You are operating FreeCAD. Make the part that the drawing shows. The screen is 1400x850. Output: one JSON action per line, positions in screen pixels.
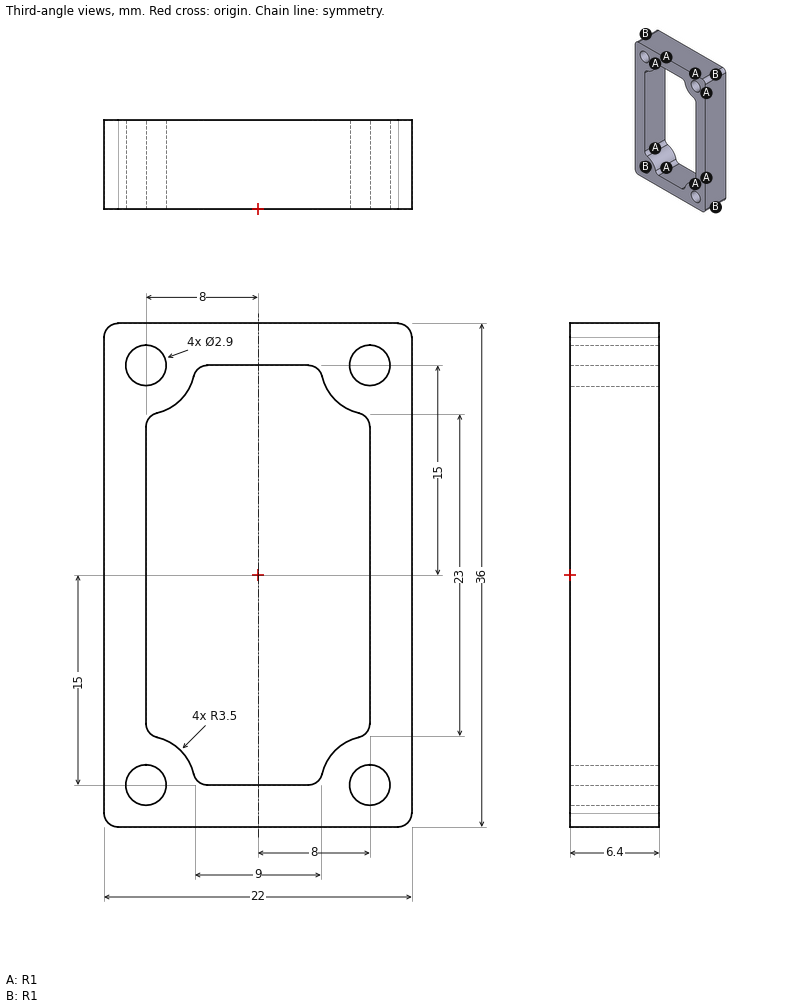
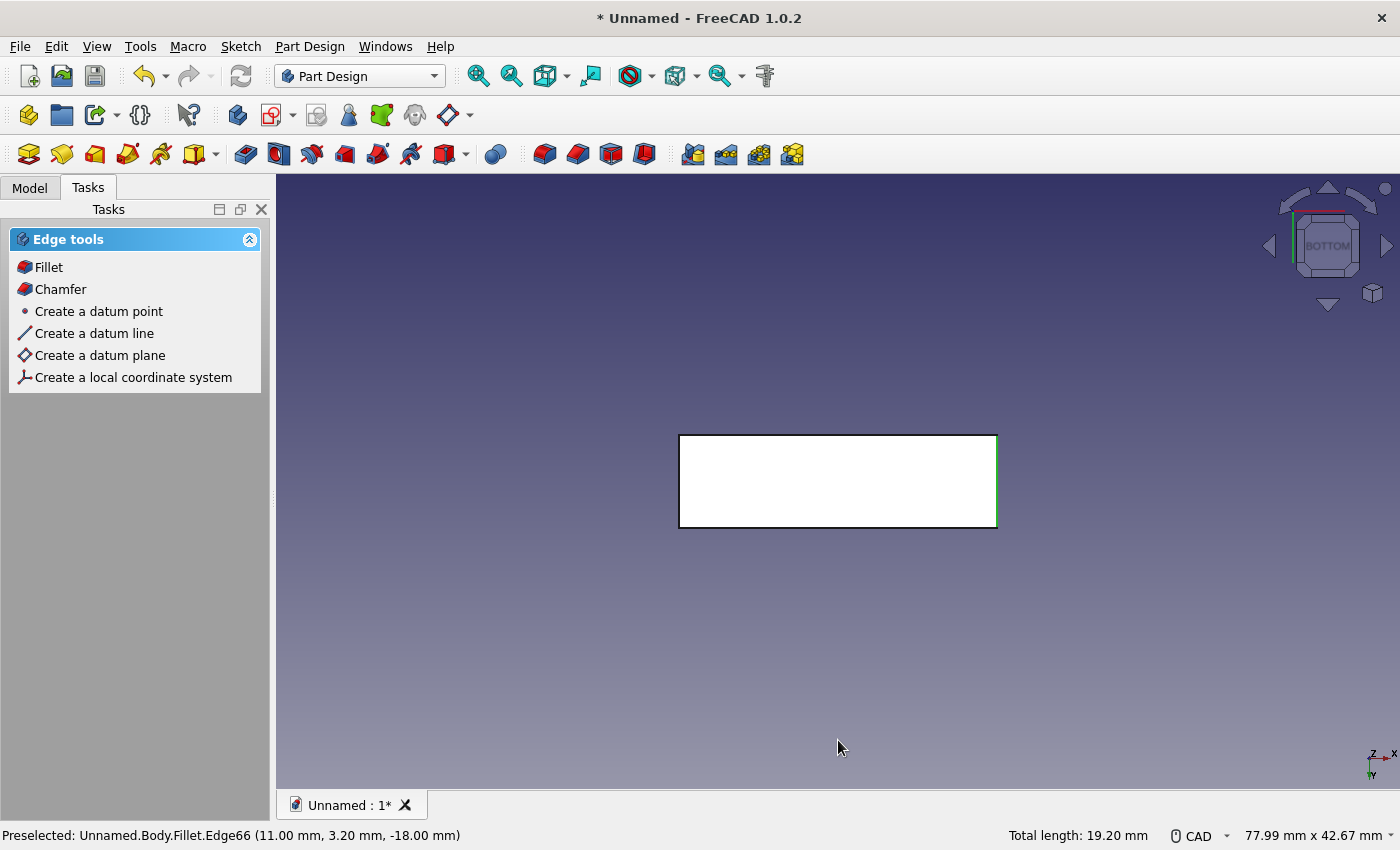
{"action": "left_click", "coordinate": [479, 76]}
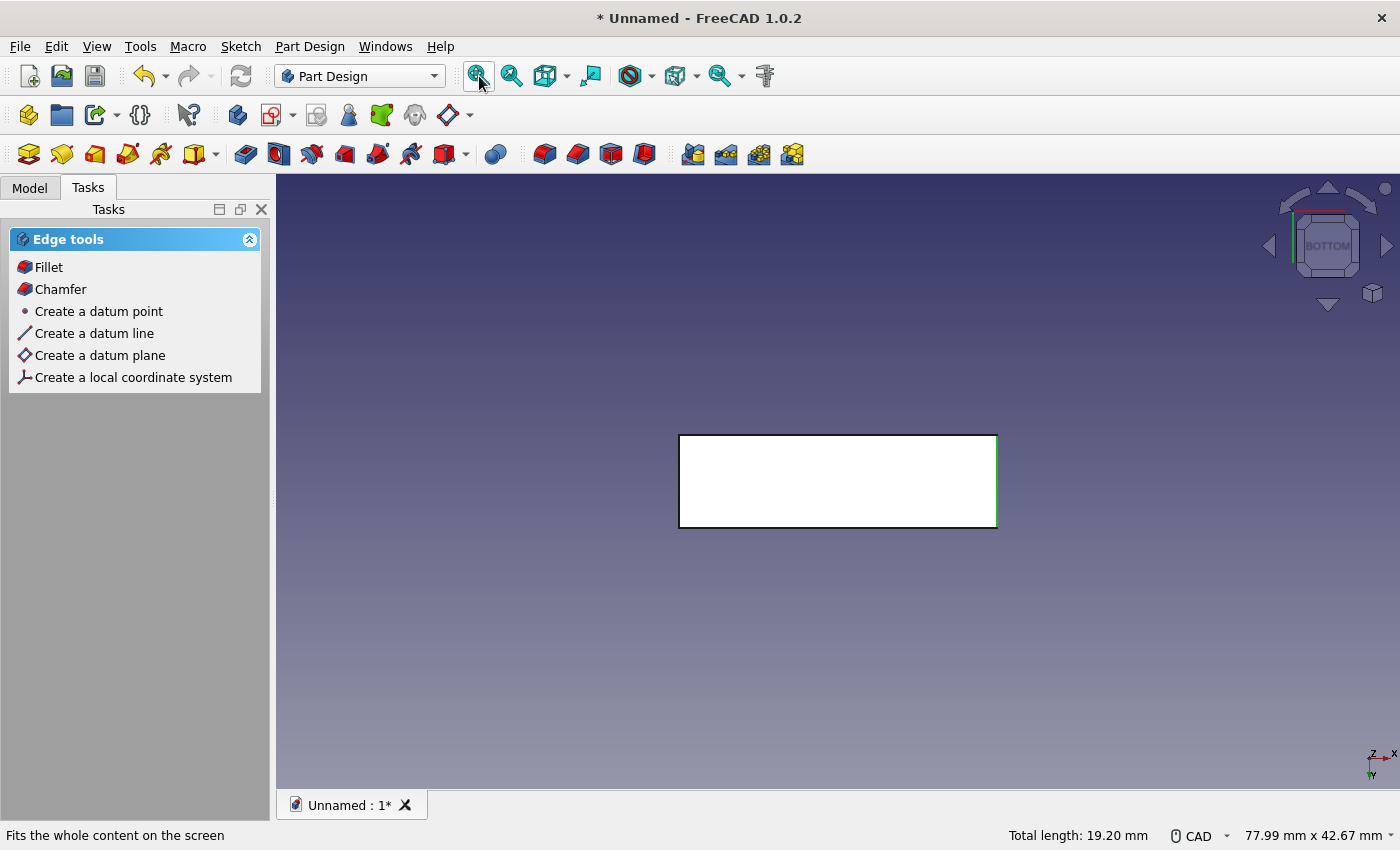
{"action": "left_click", "coordinate": [679, 480], "text": "ctrl"}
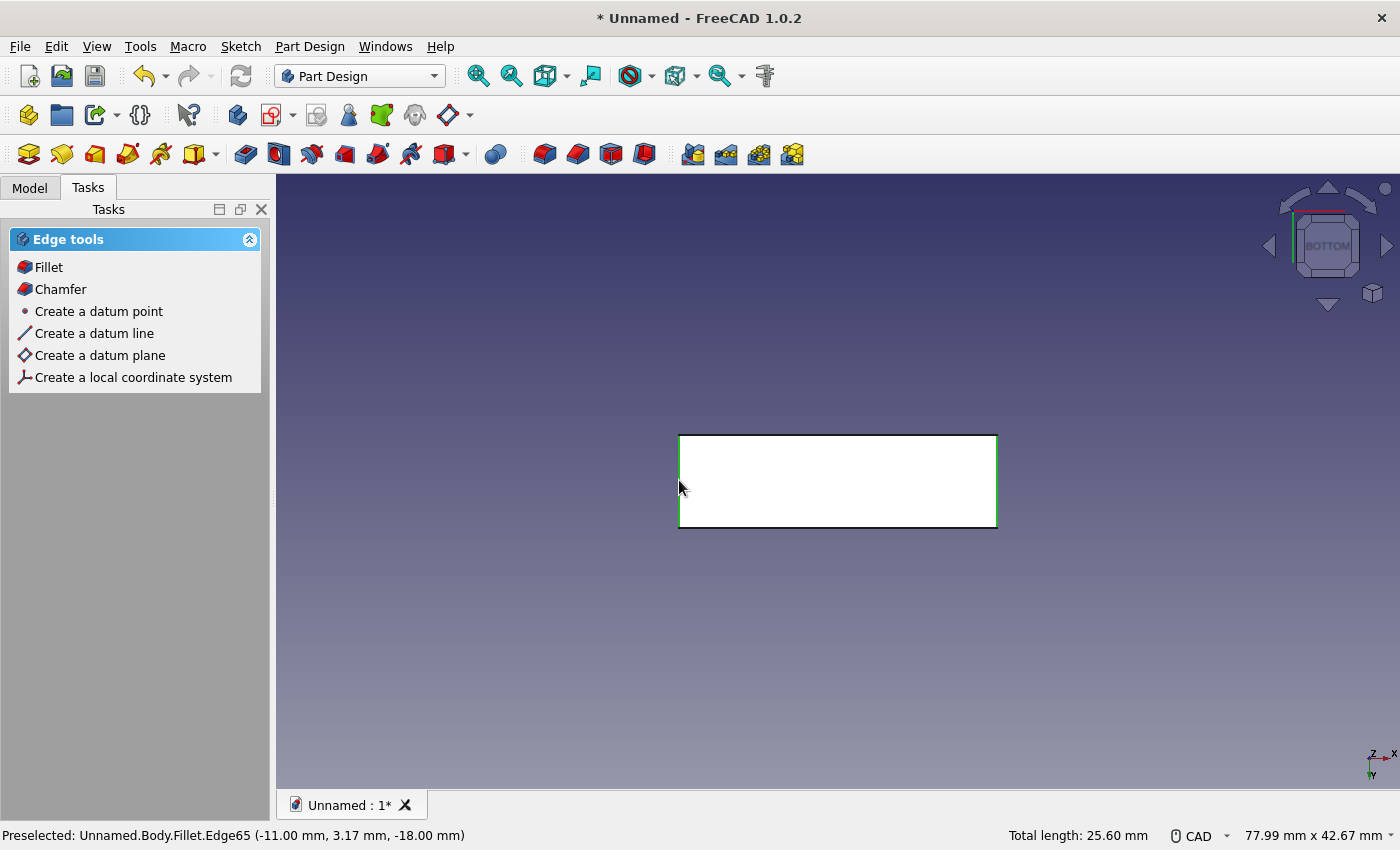
{"action": "left_click", "coordinate": [545, 154]}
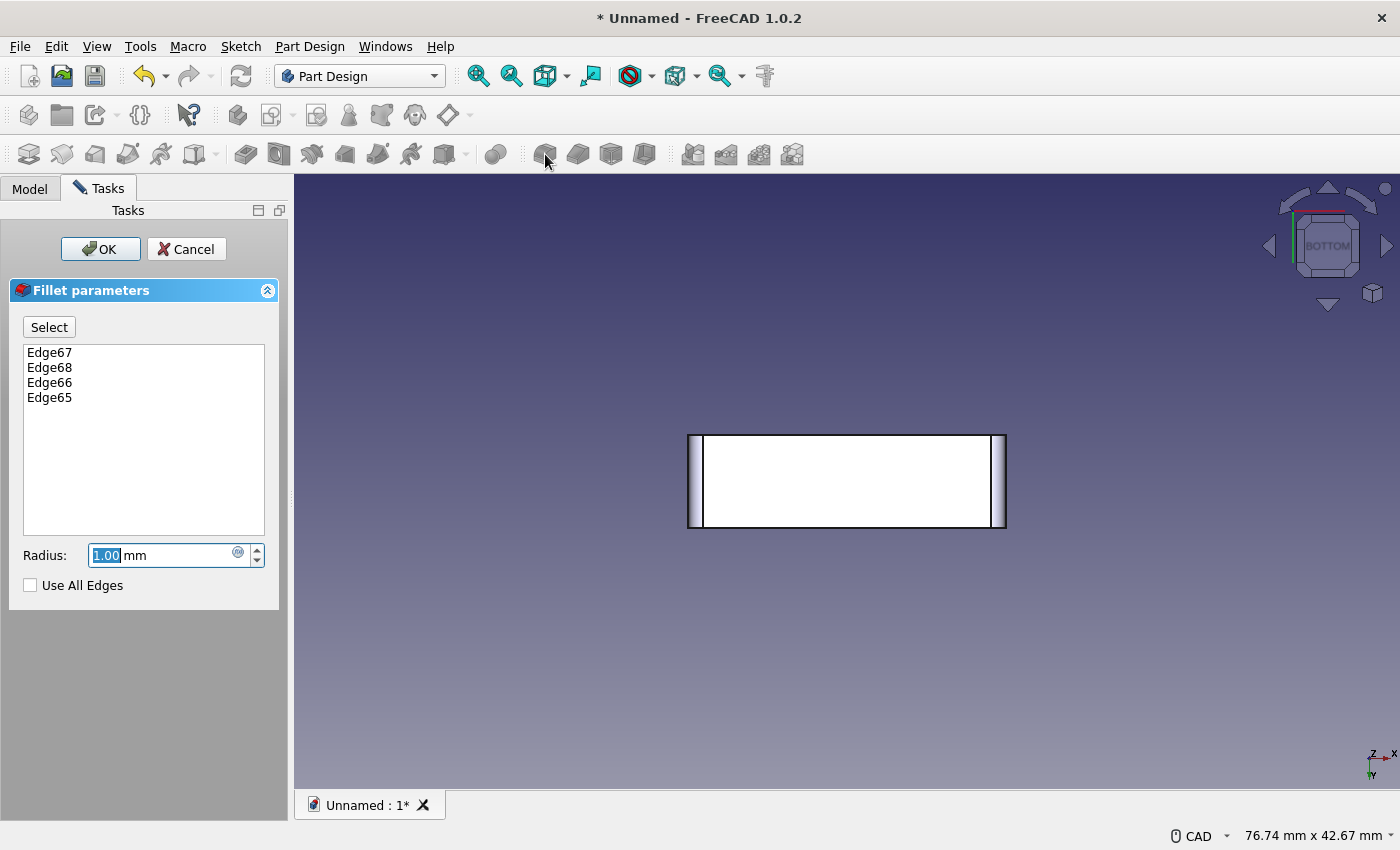
{"action": "type", "text": "1"}
{"action": "key", "text": "Tab"}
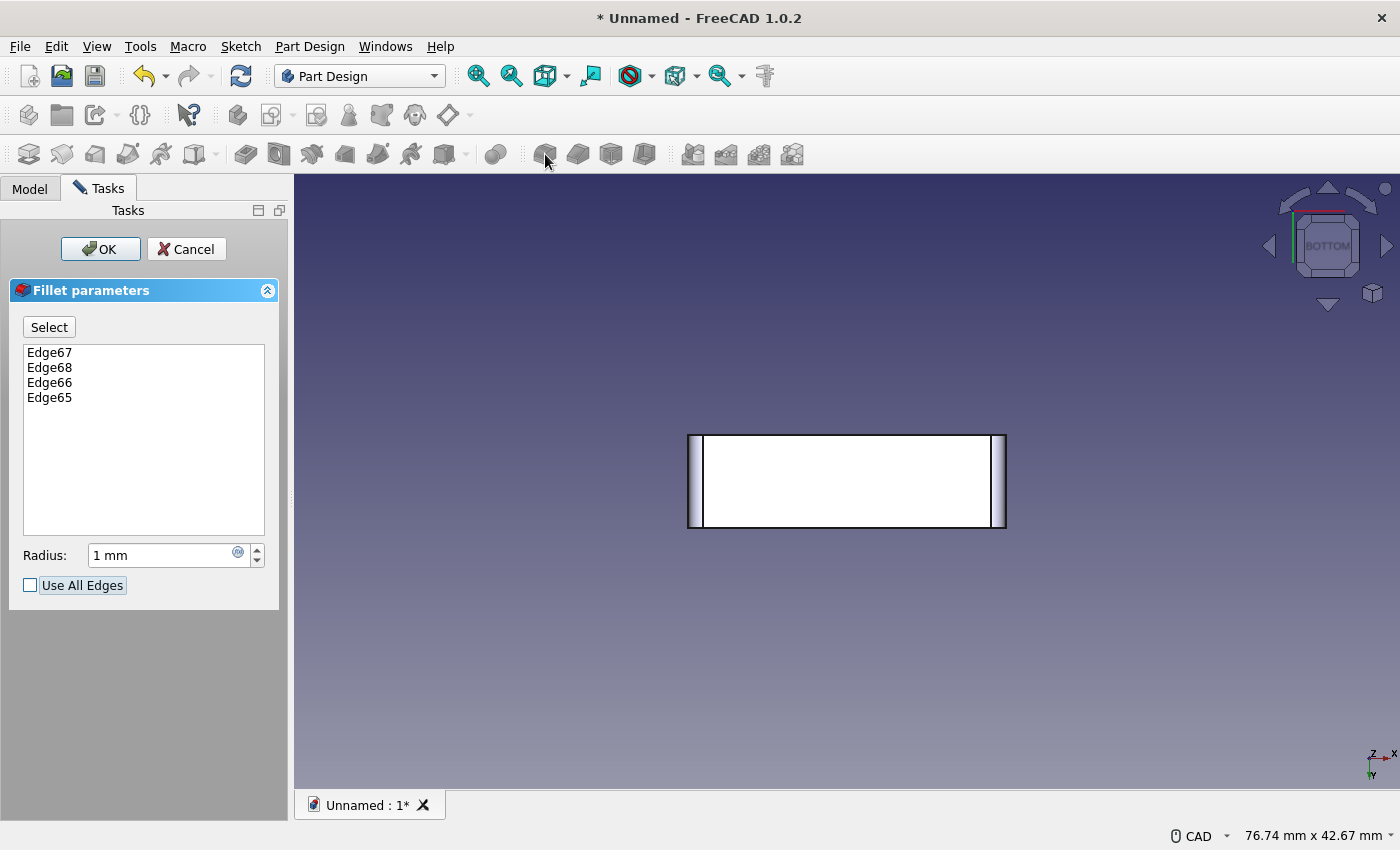
{"action": "left_click", "coordinate": [101, 249]}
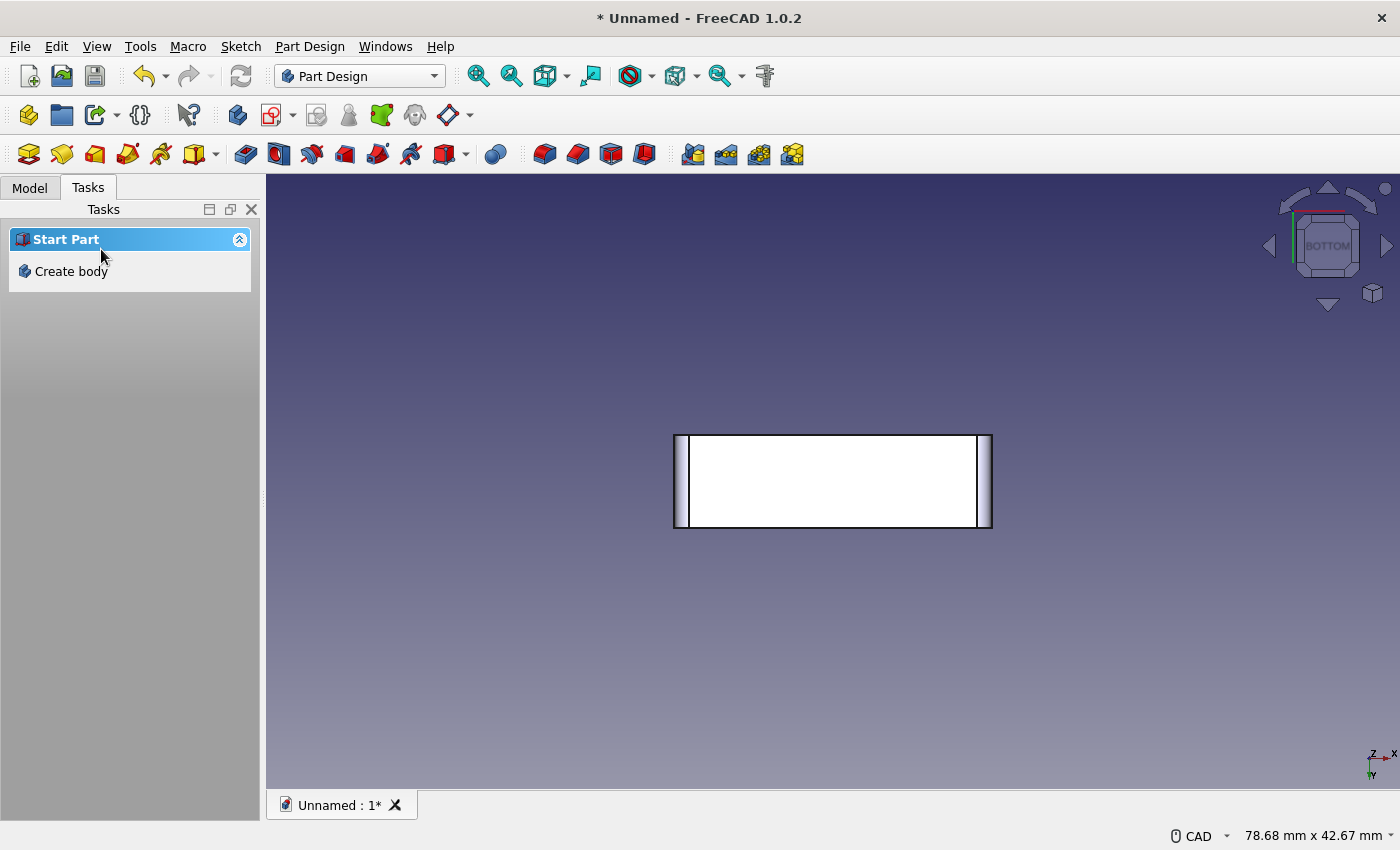
{"action": "key", "text": "0"}